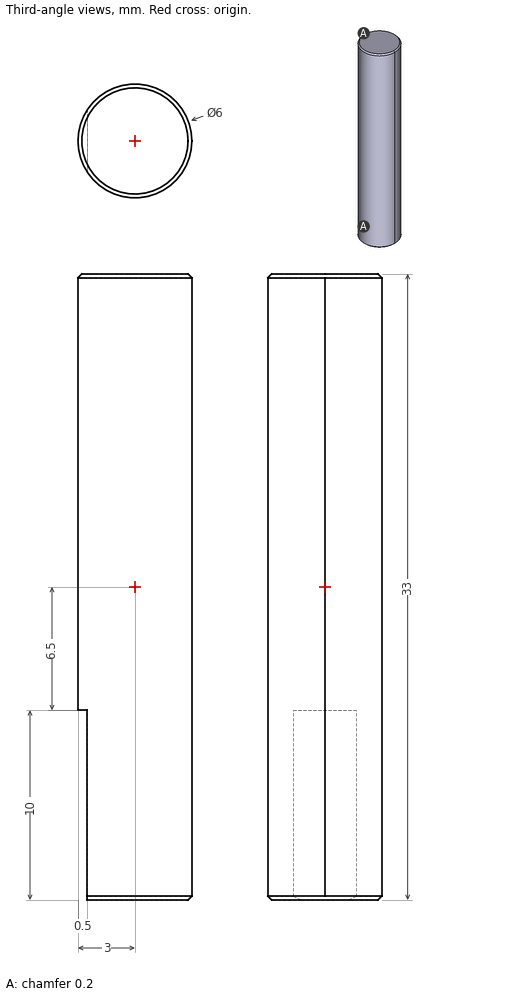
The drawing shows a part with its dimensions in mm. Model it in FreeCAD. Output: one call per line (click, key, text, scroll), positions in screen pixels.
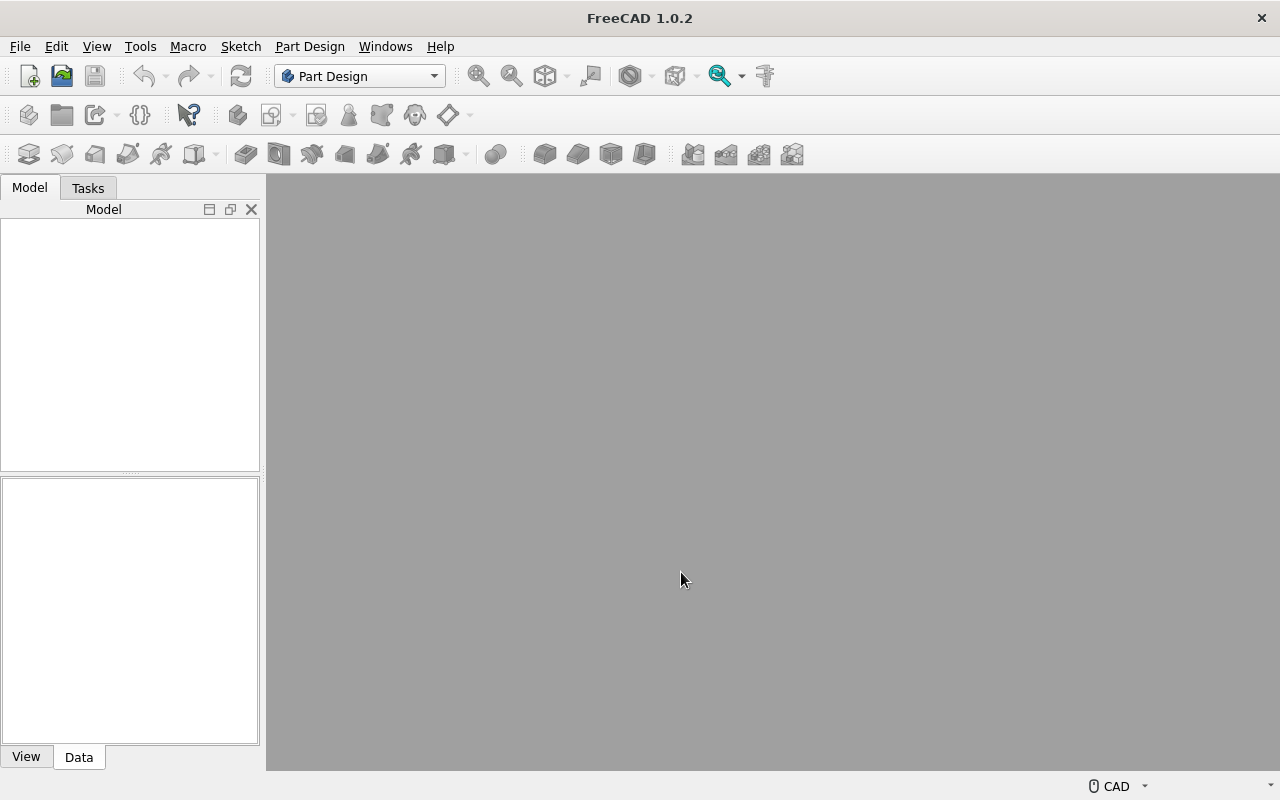
click(29, 76)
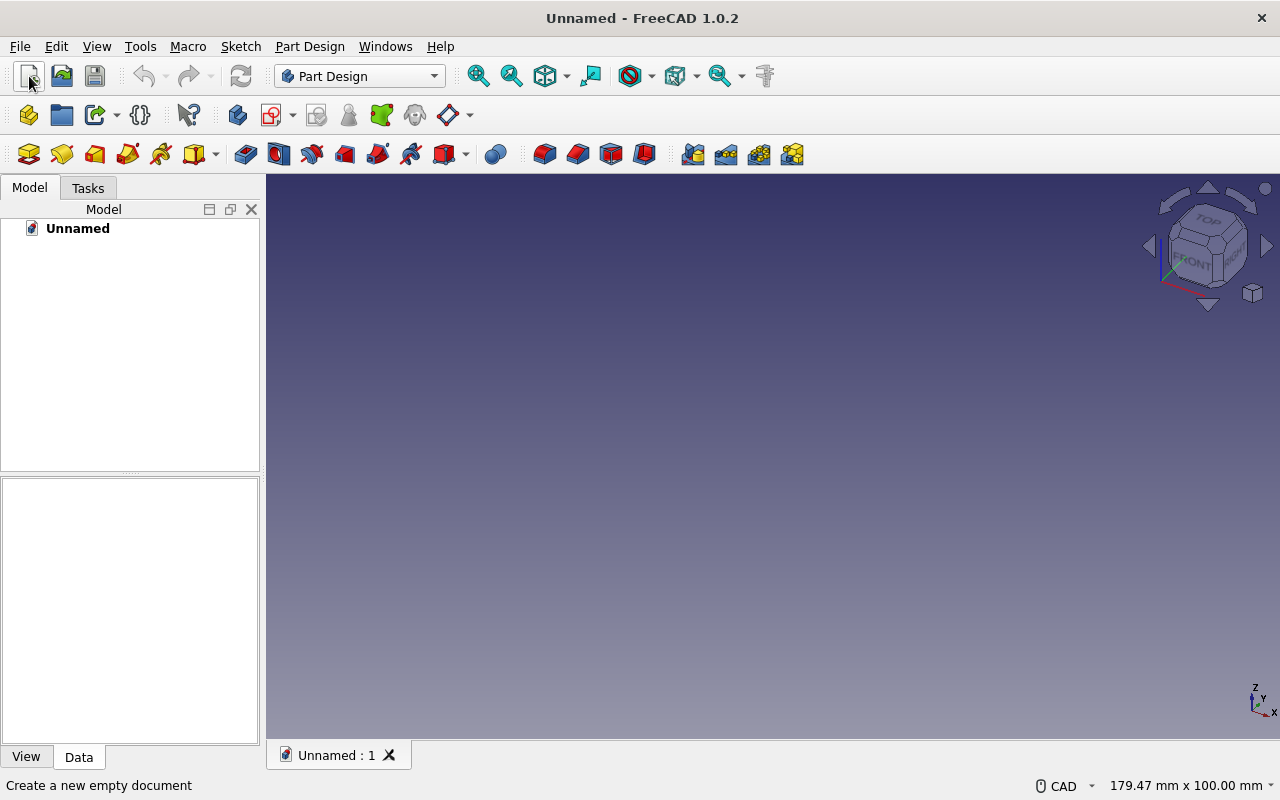
click(270, 116)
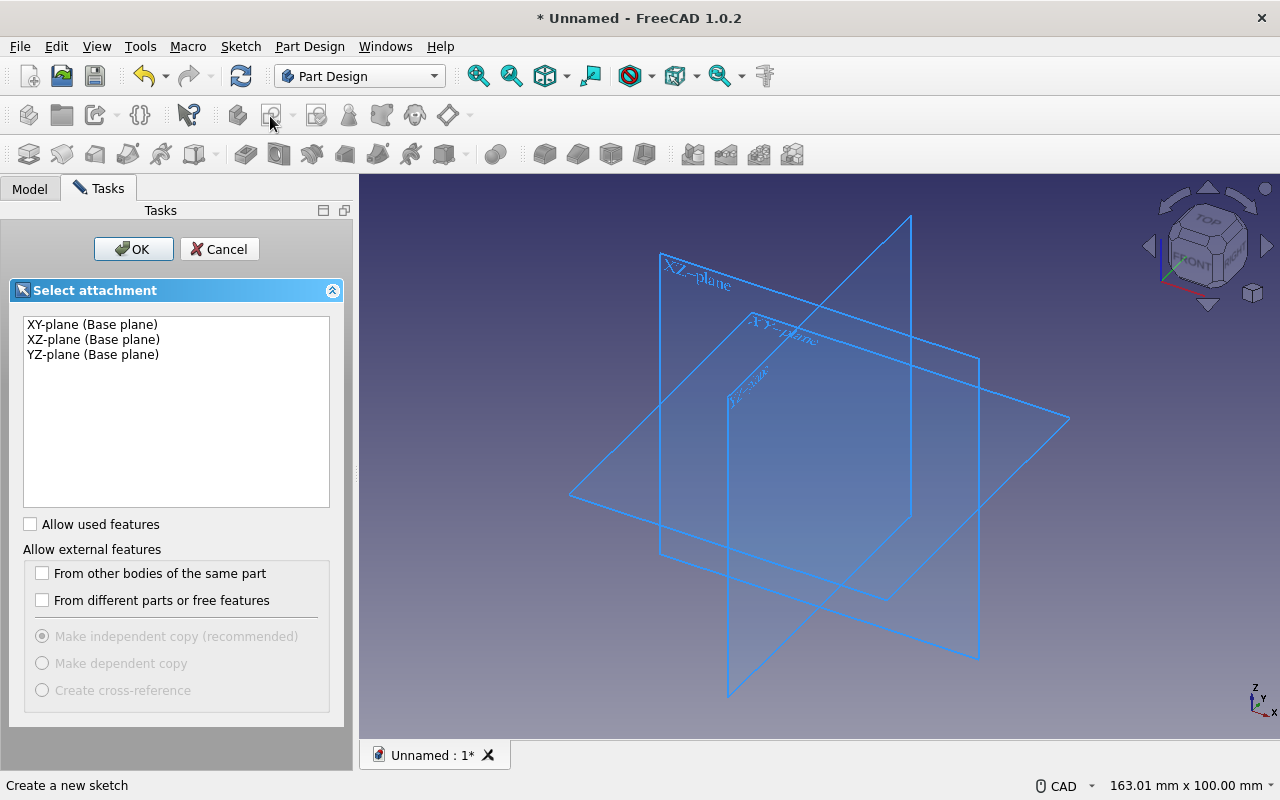
click(84, 324)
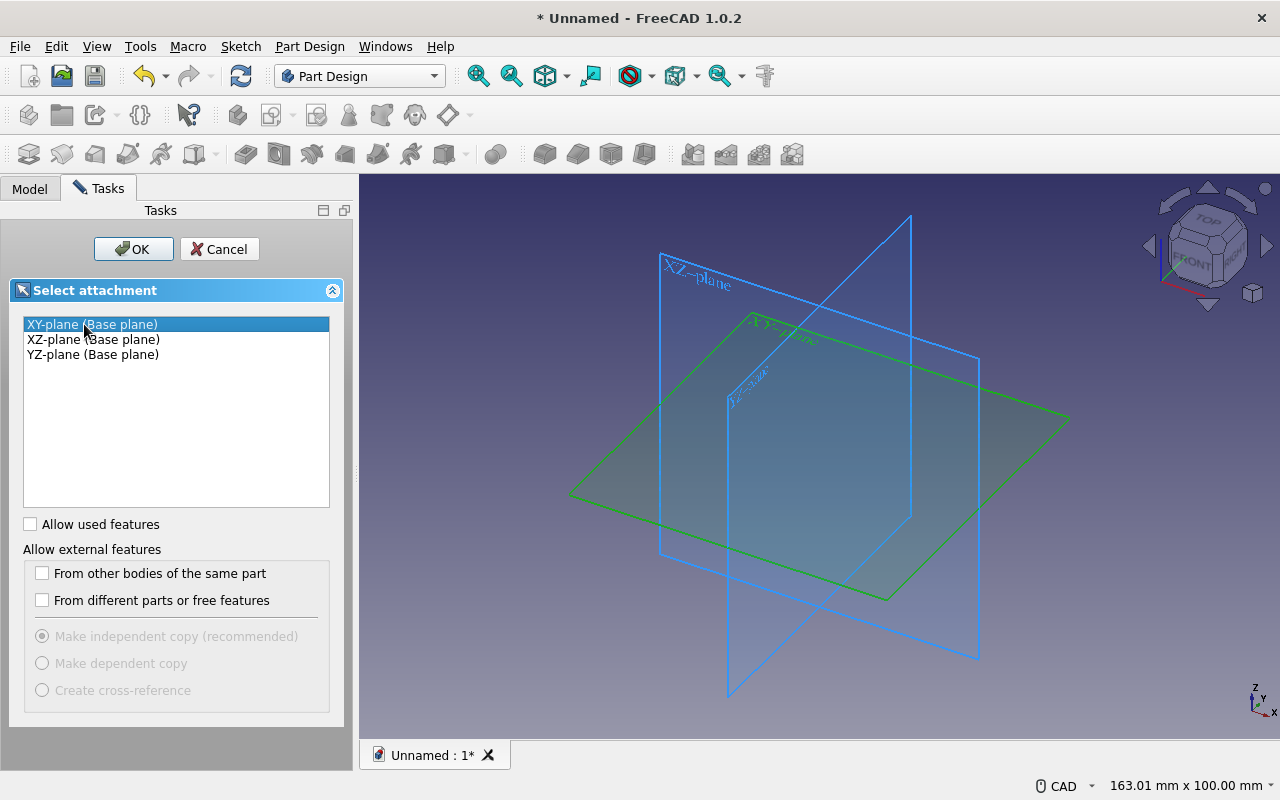
click(134, 249)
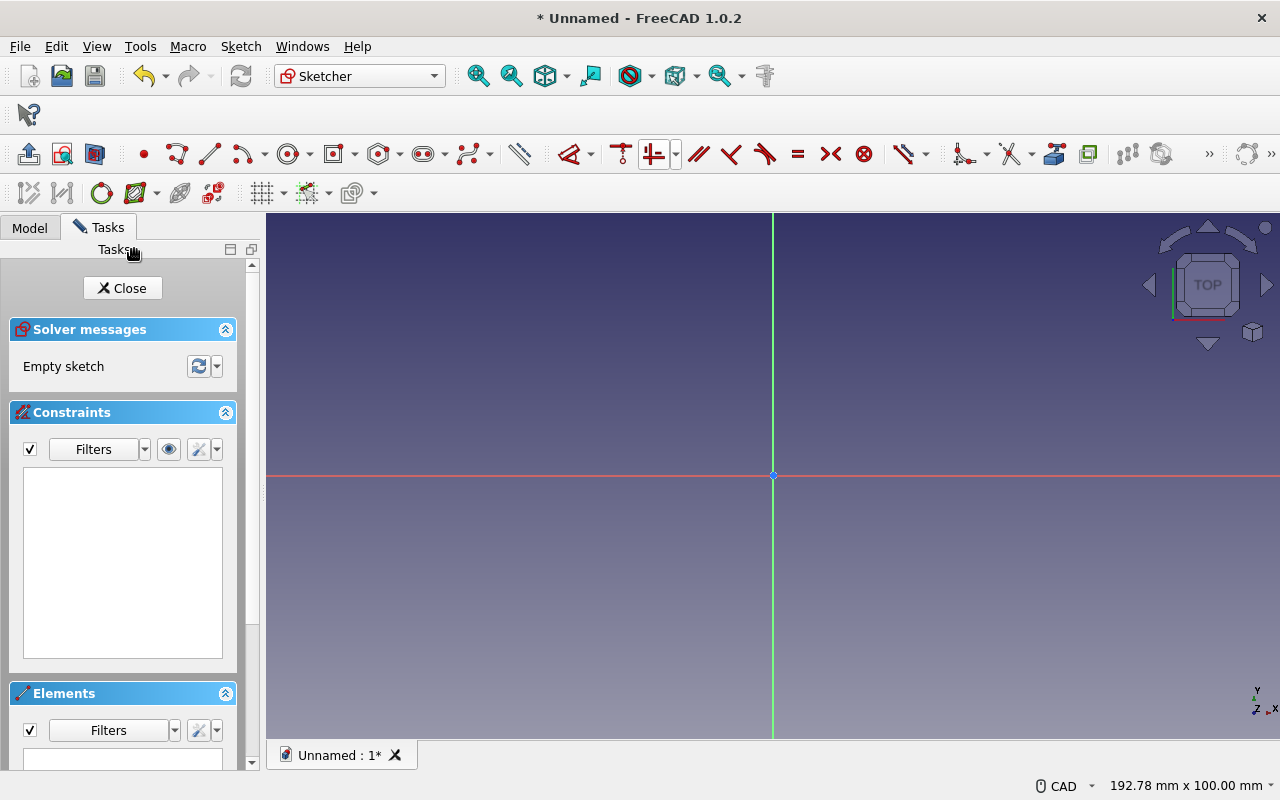
scroll(780, 476, up, 12)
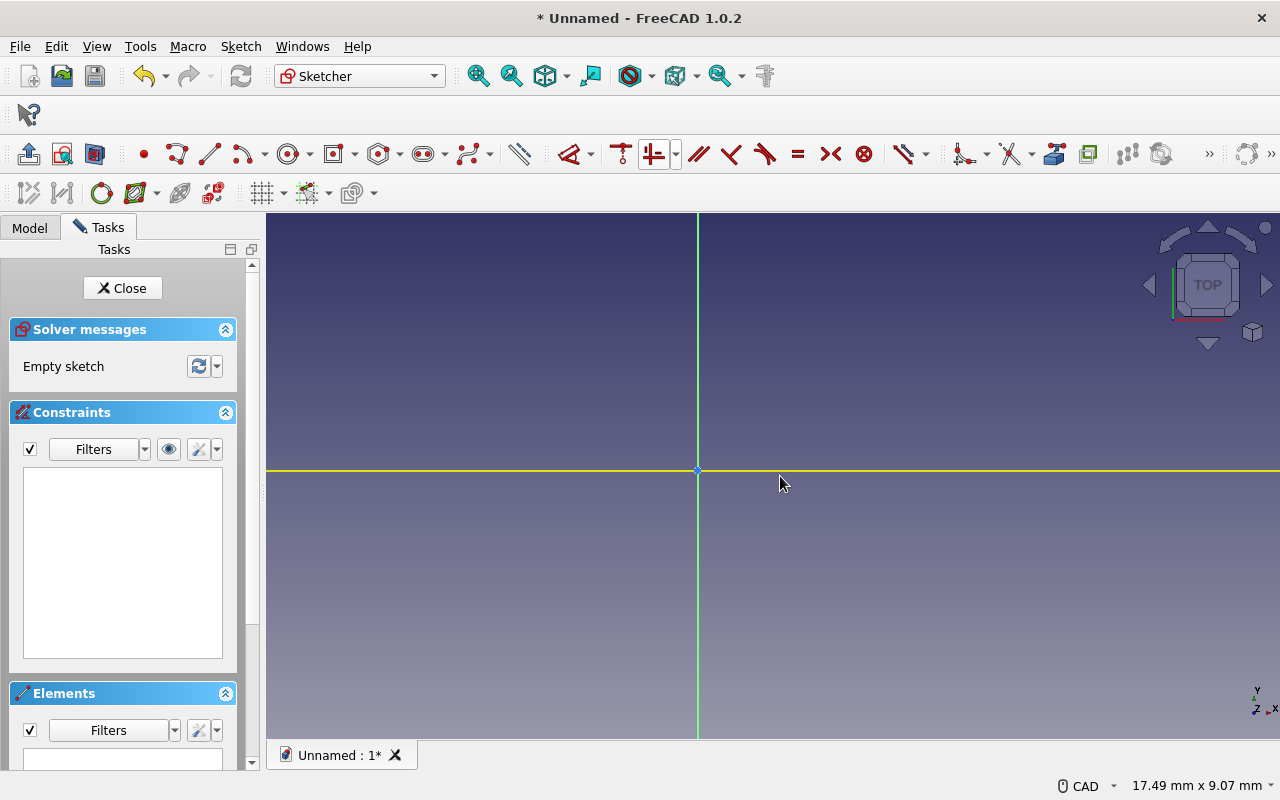
key(g)
key(c)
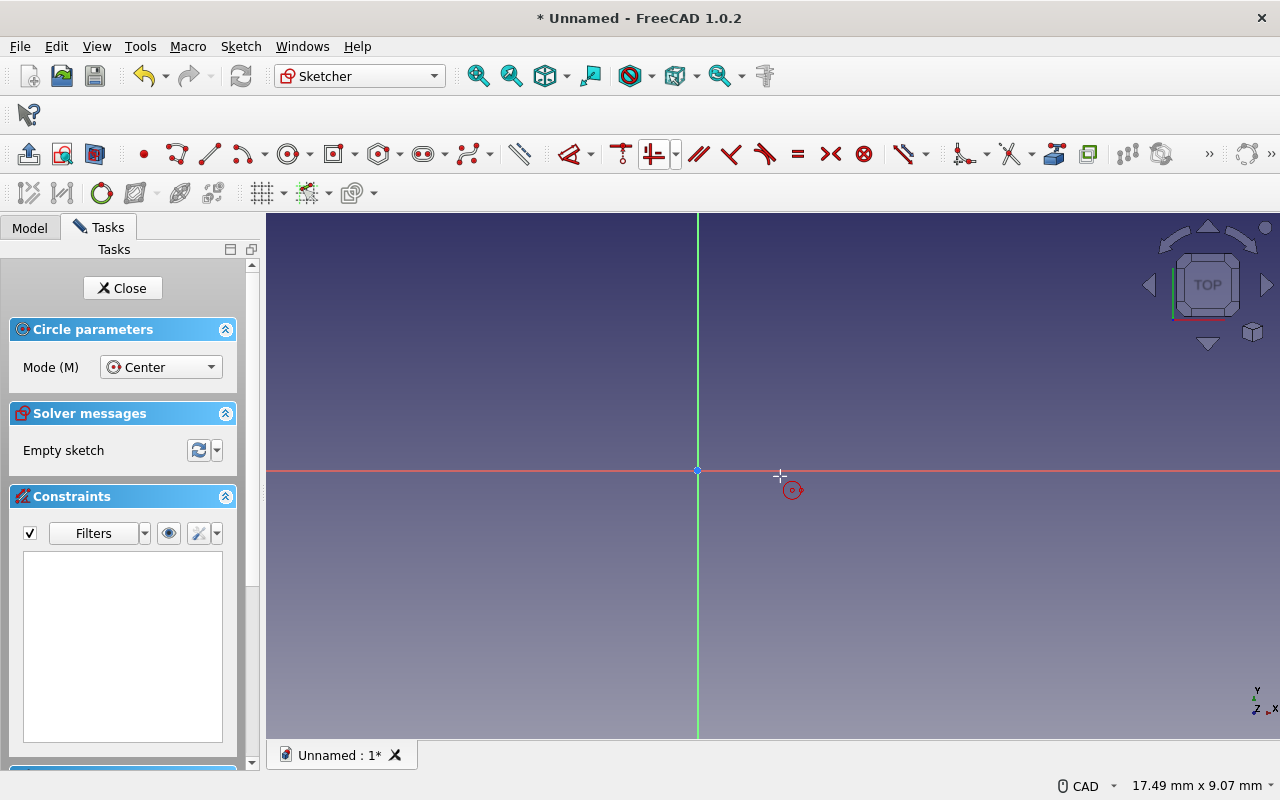
click(698, 471)
move(821, 348)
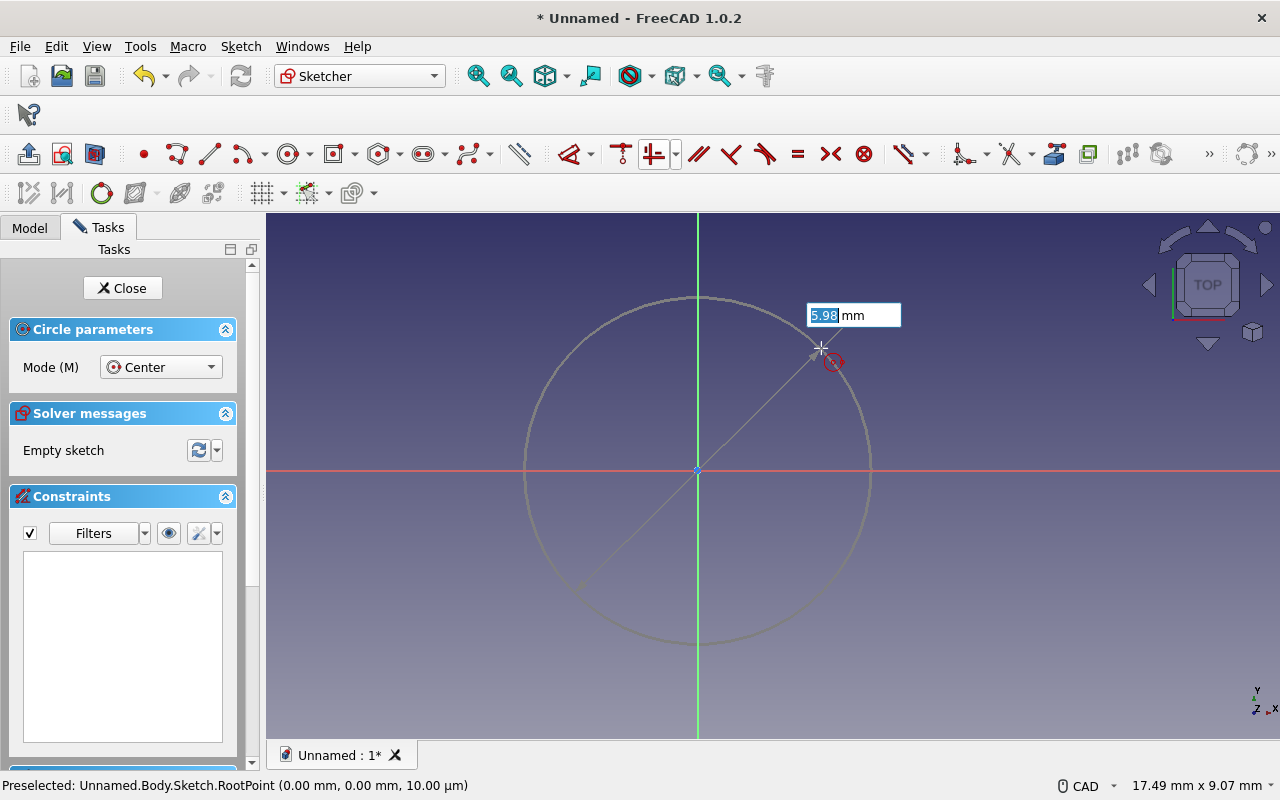
text(6)
key(Return)
key(Escape)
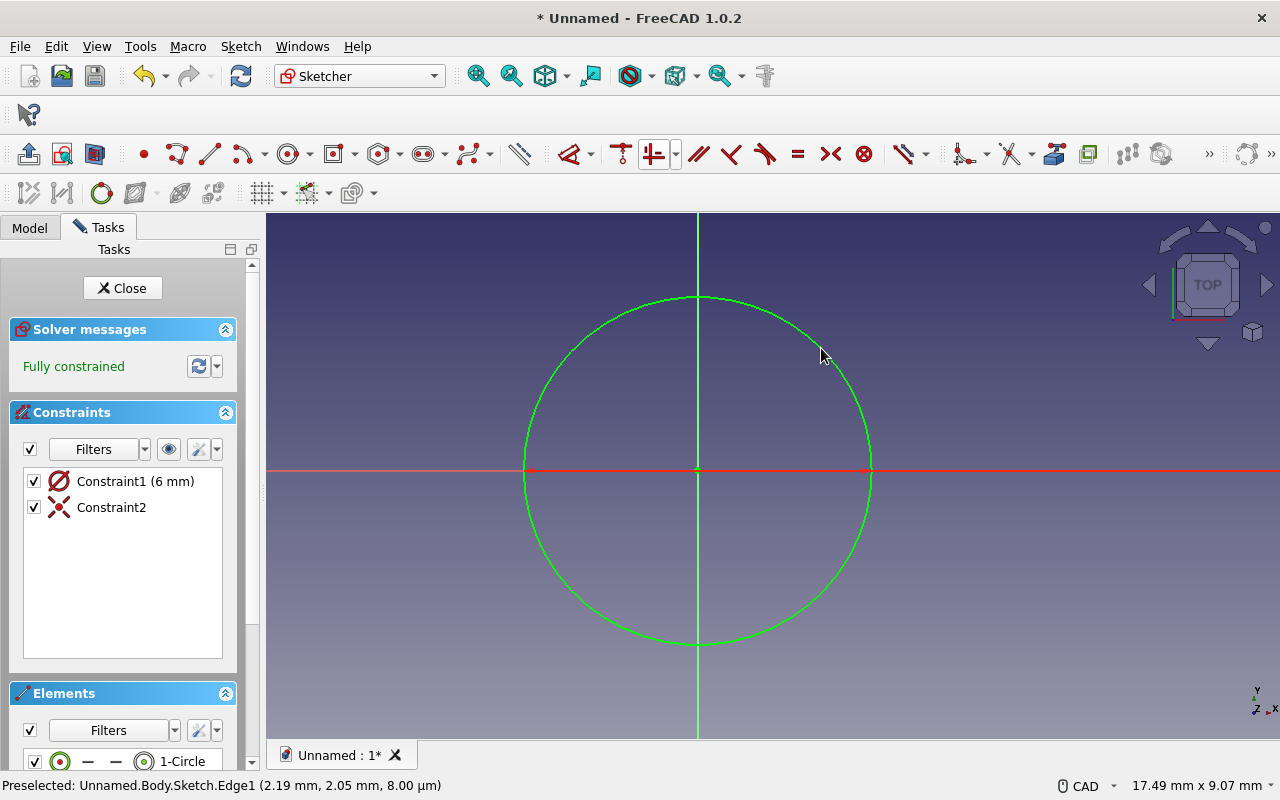
click(123, 288)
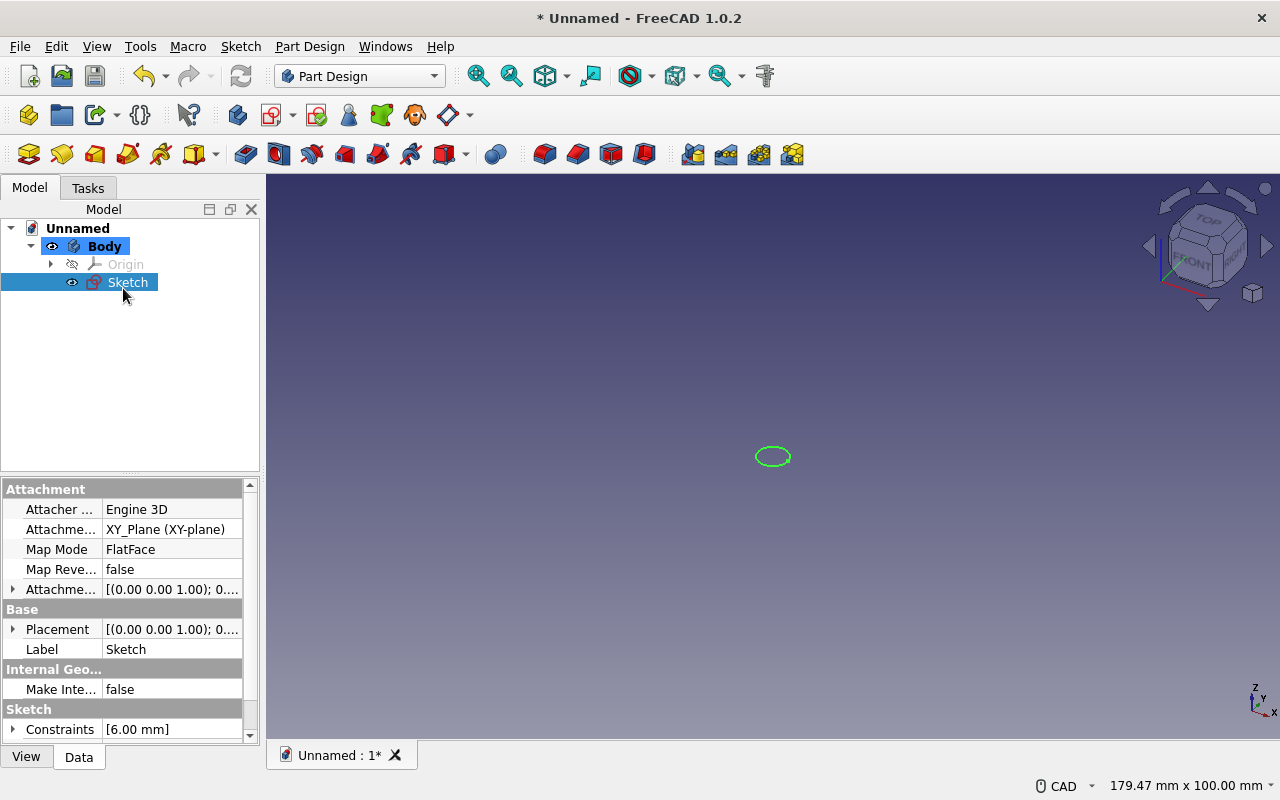
click(29, 154)